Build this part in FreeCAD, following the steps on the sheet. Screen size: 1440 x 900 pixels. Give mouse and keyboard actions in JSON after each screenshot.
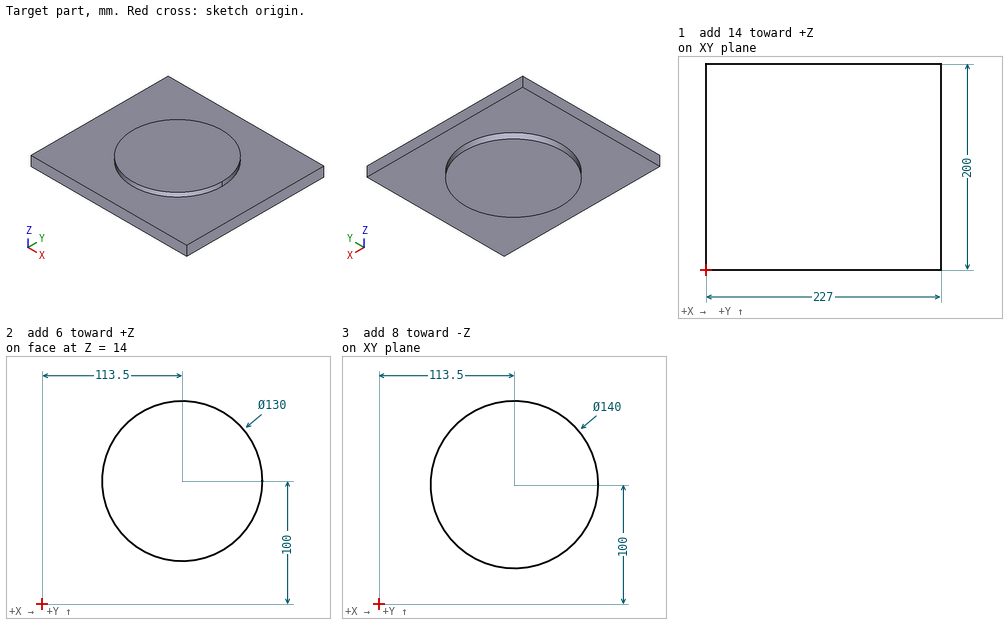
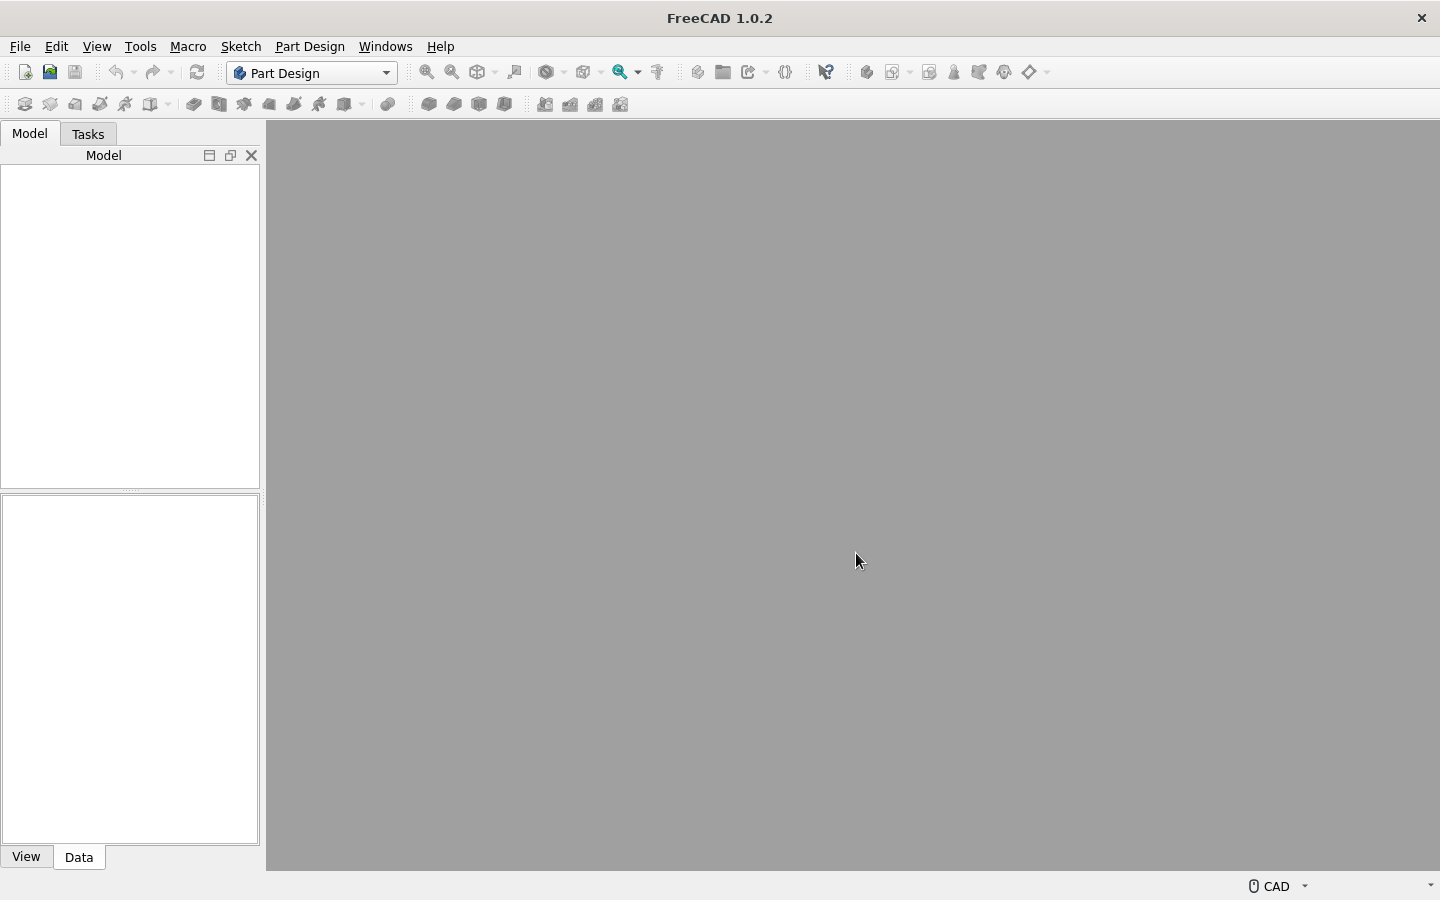
{"action": "key", "text": "ctrl+n"}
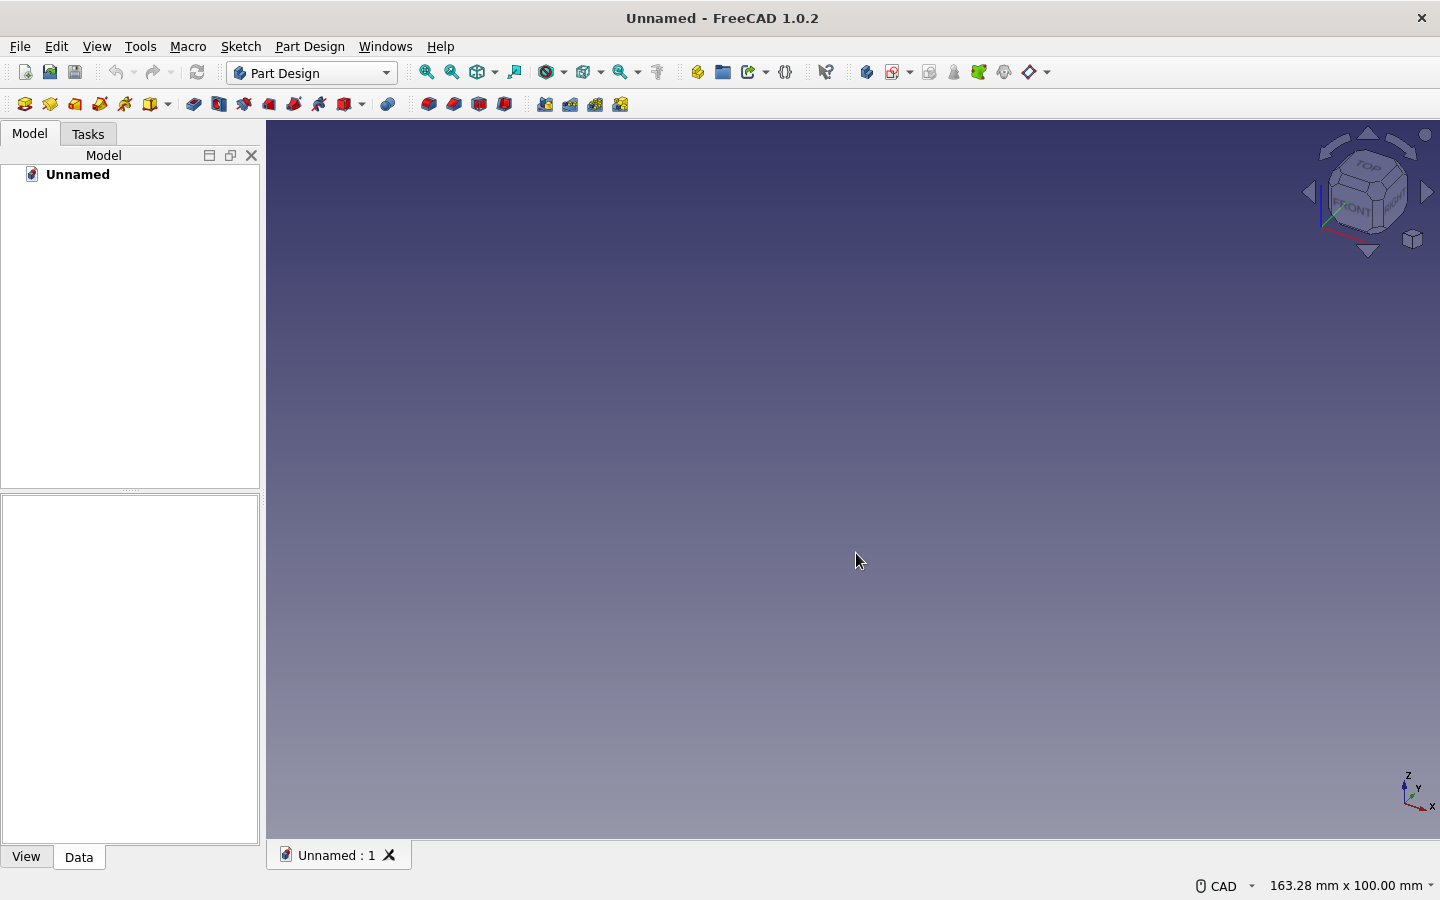
{"action": "left_click", "coordinate": [892, 72]}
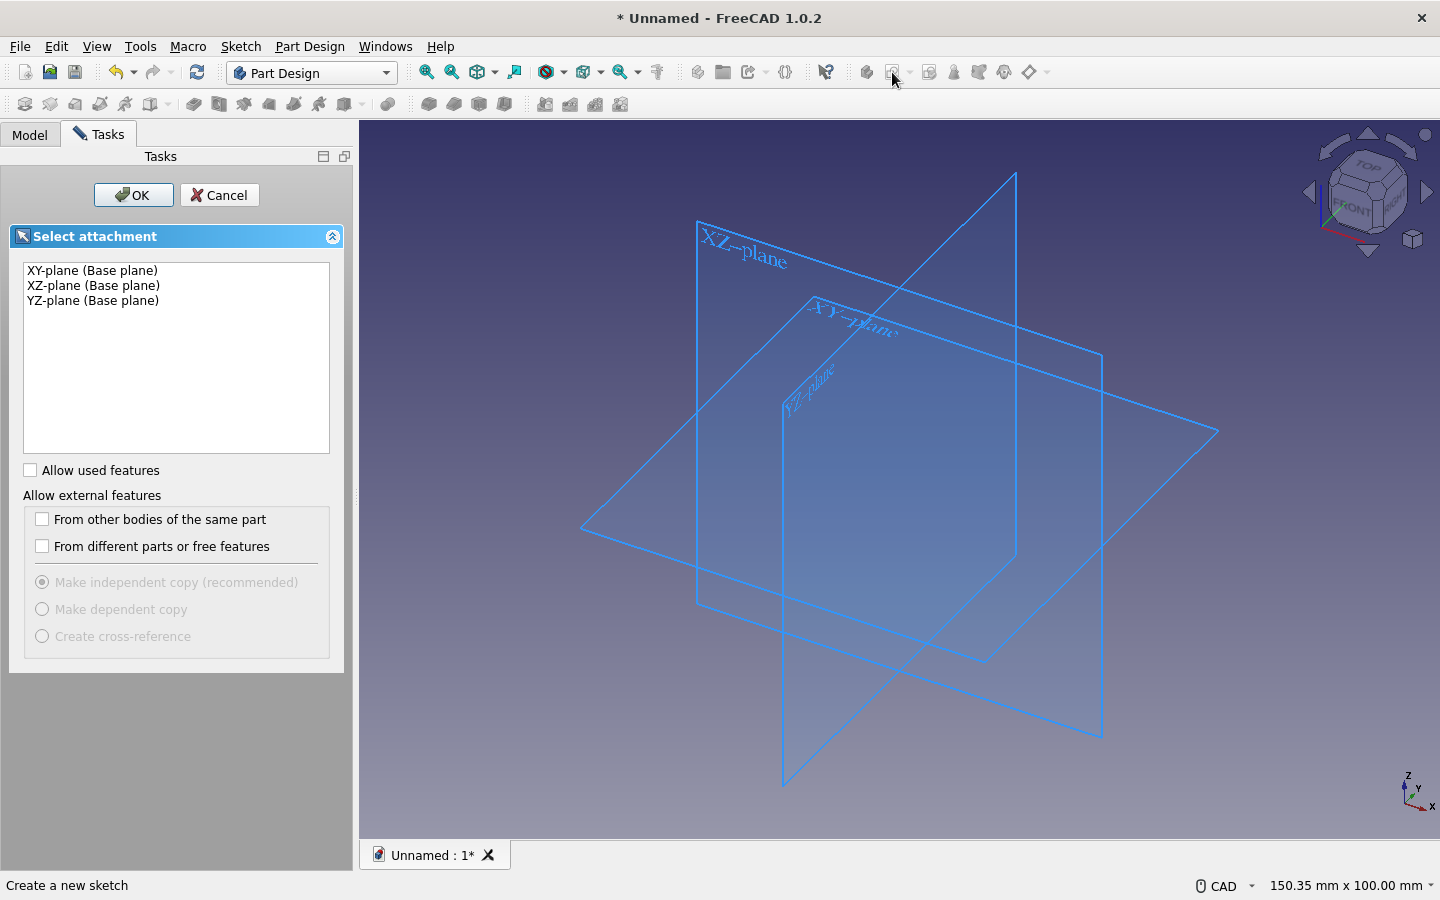
{"action": "left_click", "coordinate": [84, 270]}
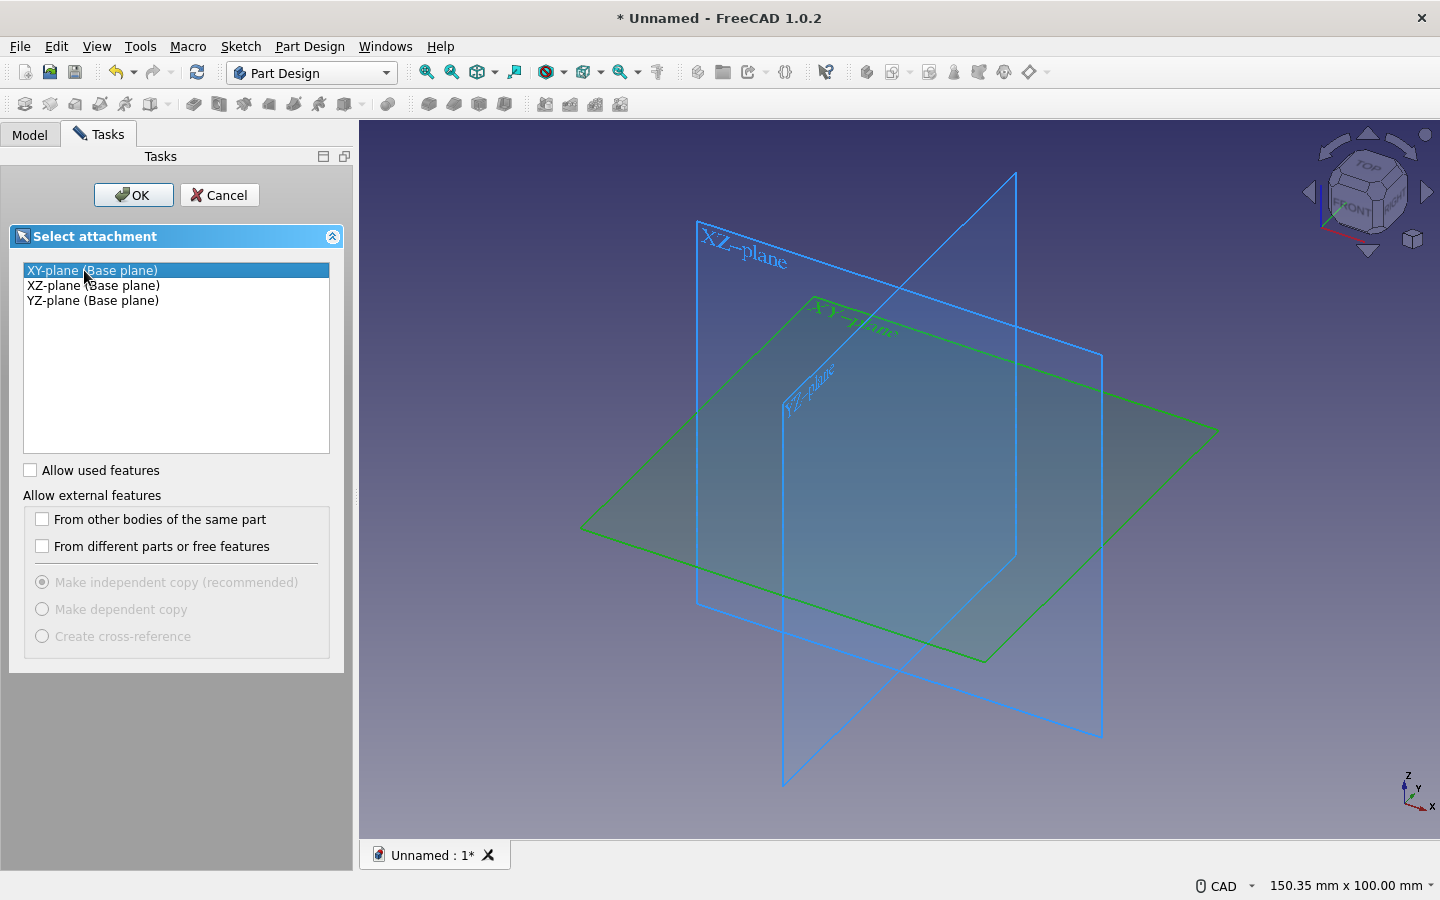
{"action": "left_click", "coordinate": [134, 195]}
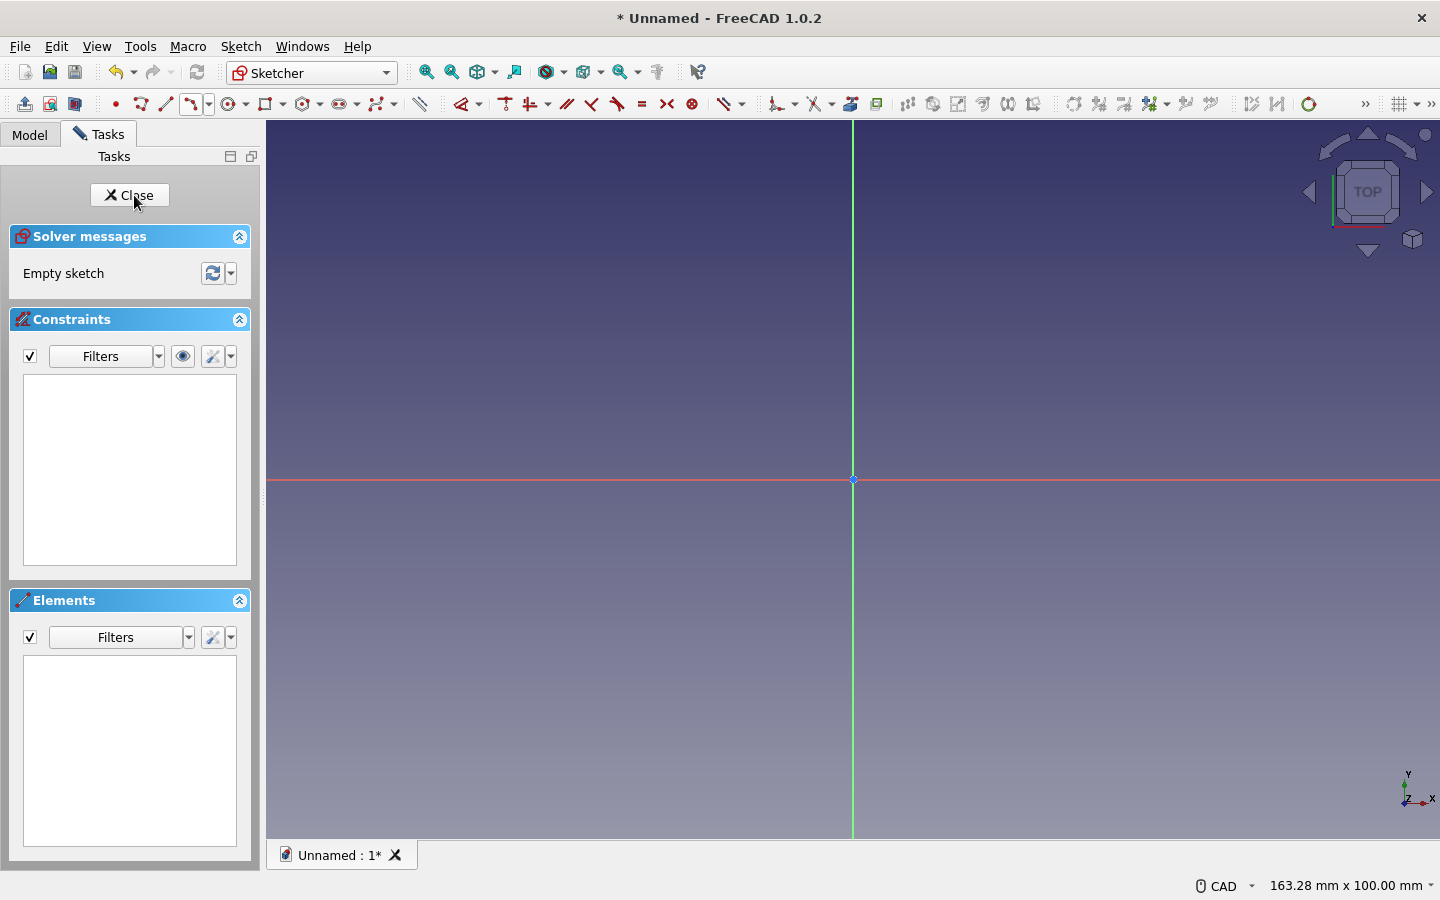
{"action": "scroll", "coordinate": [403, 789], "scroll_direction": "down", "scroll_amount": 6}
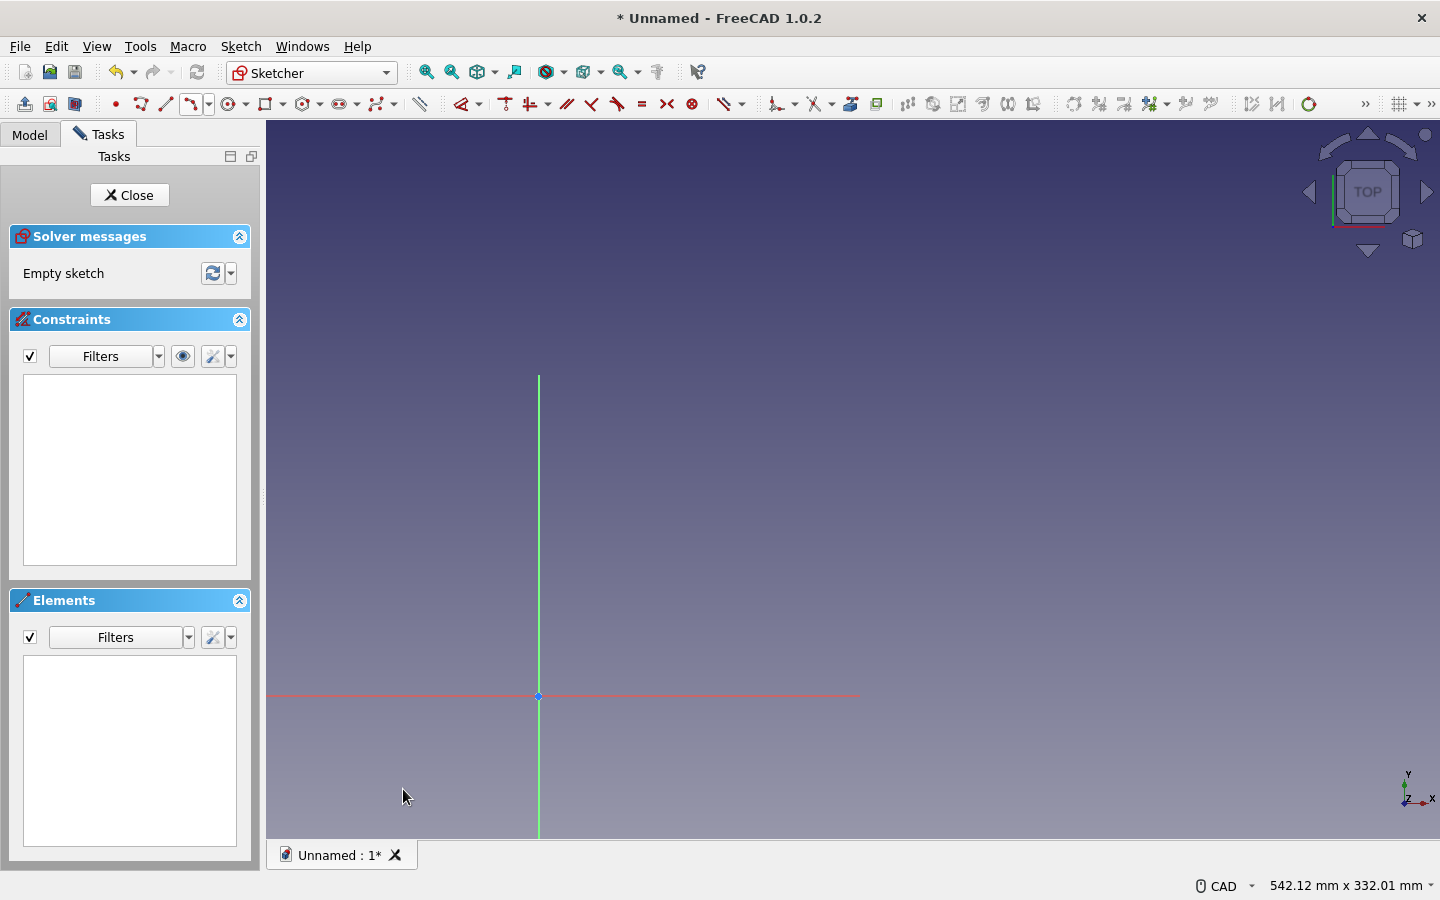
{"action": "left_click", "coordinate": [264, 104]}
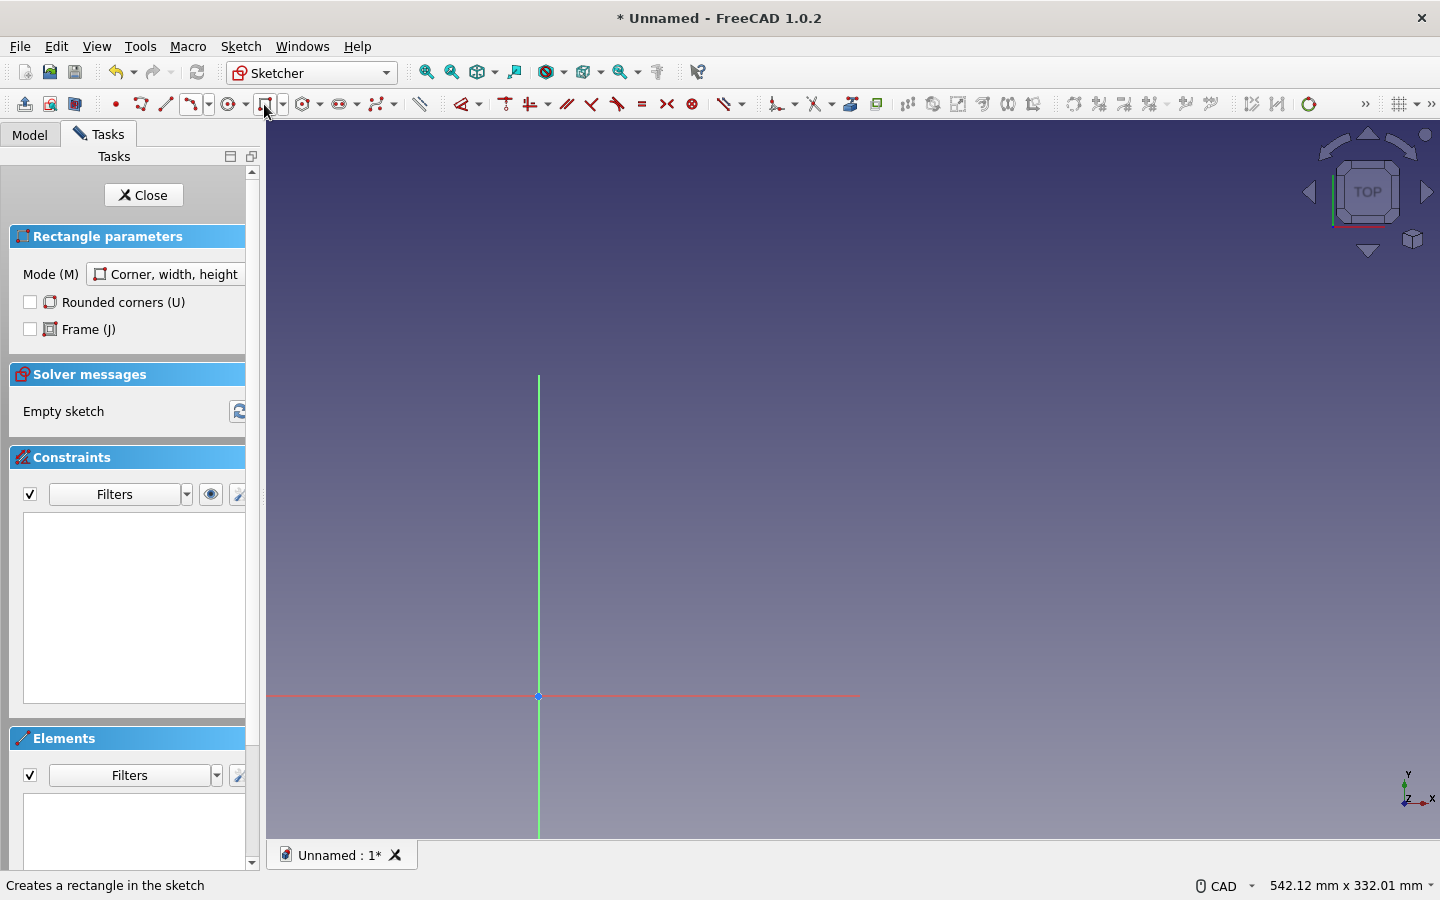
{"action": "left_click", "coordinate": [539, 696]}
{"action": "mouse_move", "coordinate": [1030, 263]}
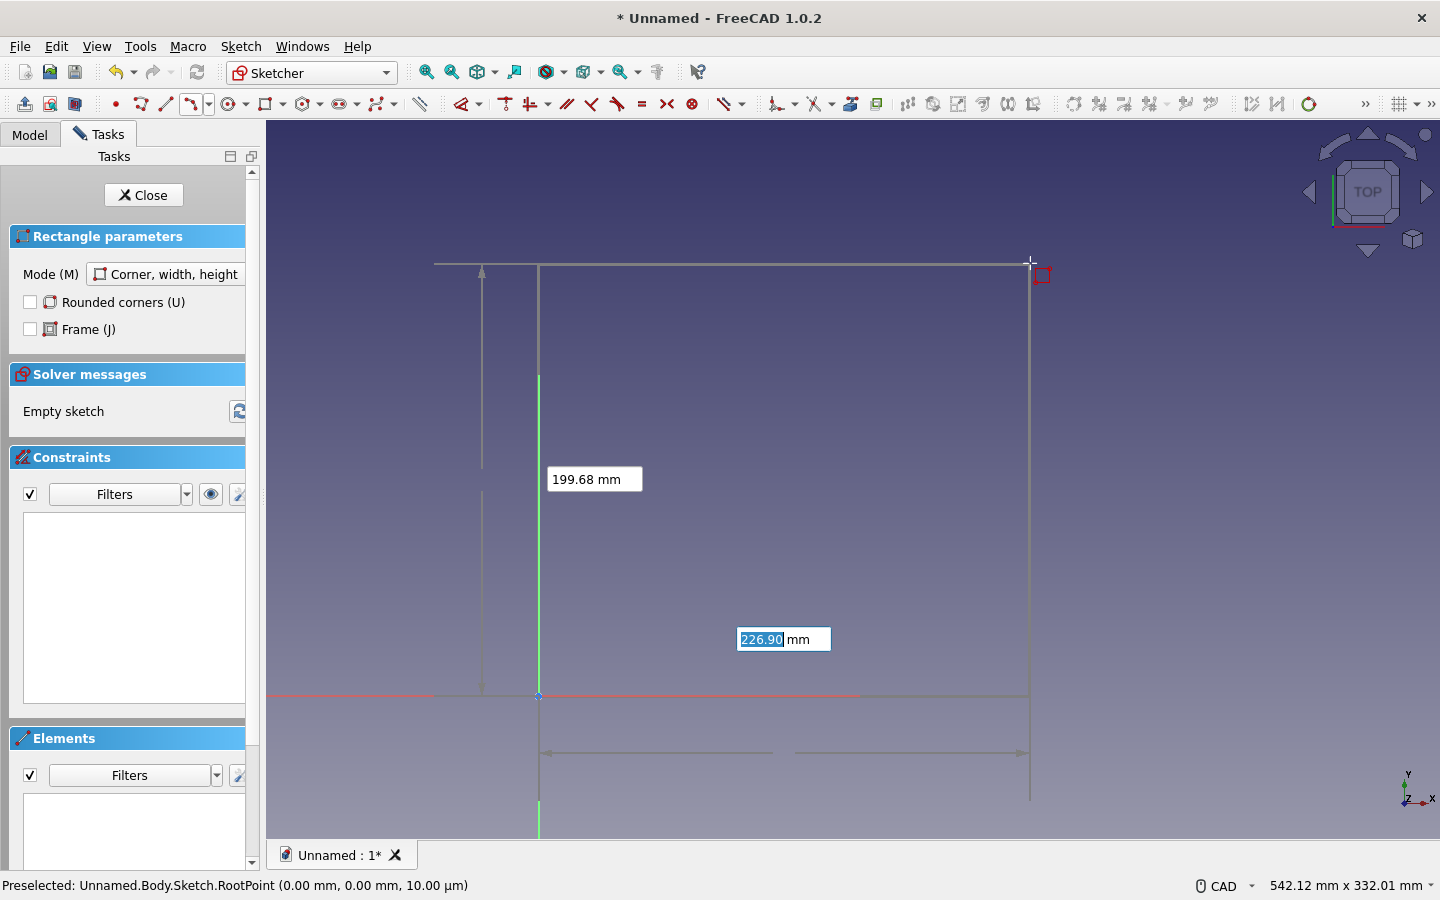
{"action": "type", "text": "227"}
{"action": "key", "text": "Tab"}
{"action": "type", "text": "200"}
{"action": "key", "text": "Return"}
{"action": "key", "text": "Escape"}